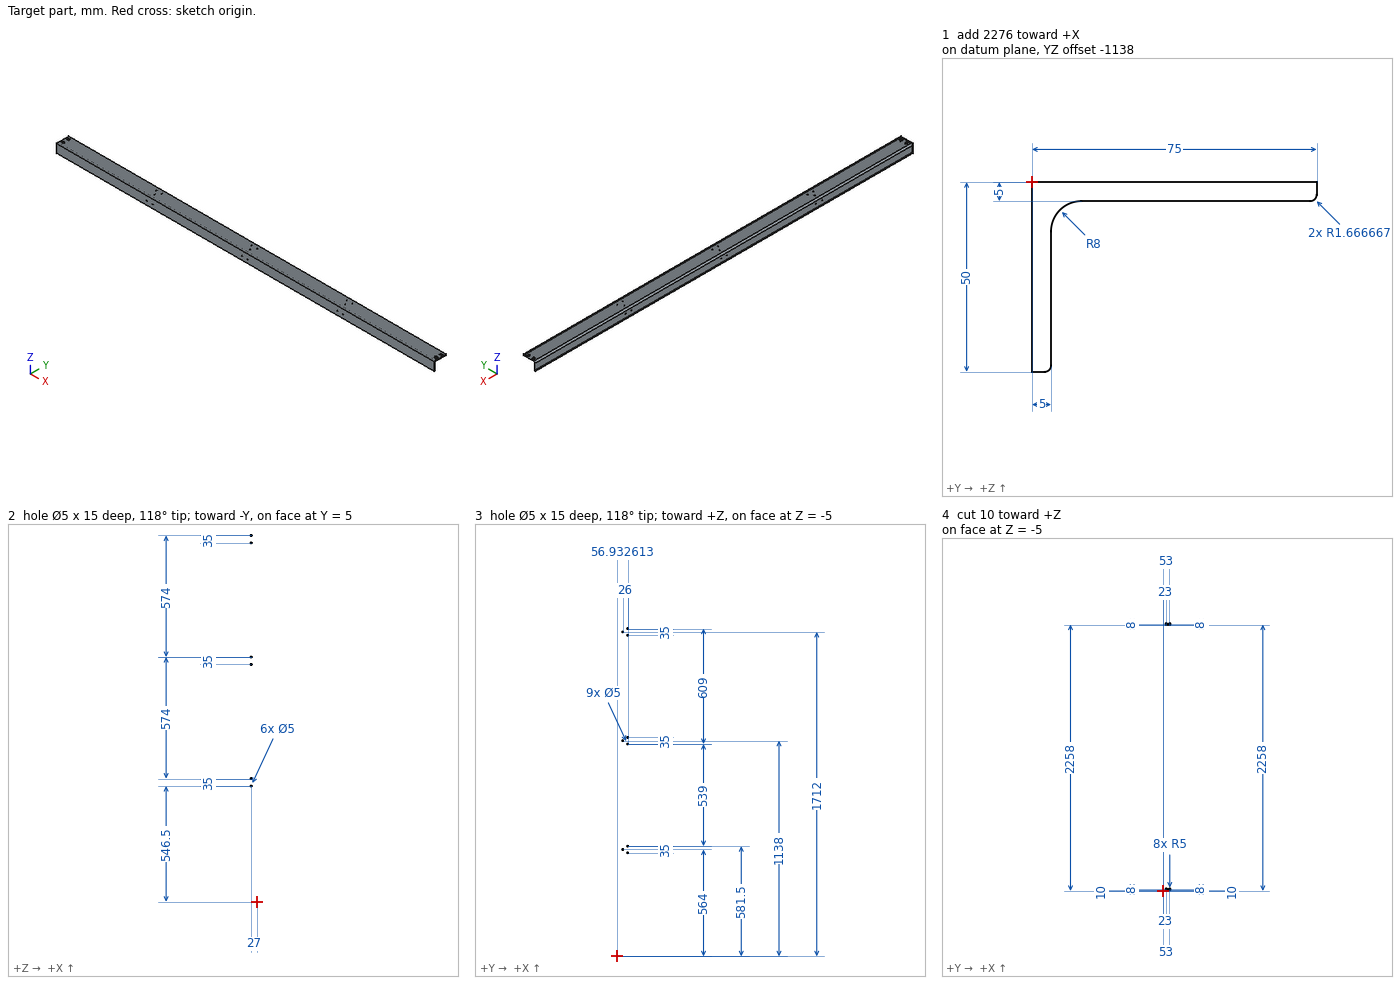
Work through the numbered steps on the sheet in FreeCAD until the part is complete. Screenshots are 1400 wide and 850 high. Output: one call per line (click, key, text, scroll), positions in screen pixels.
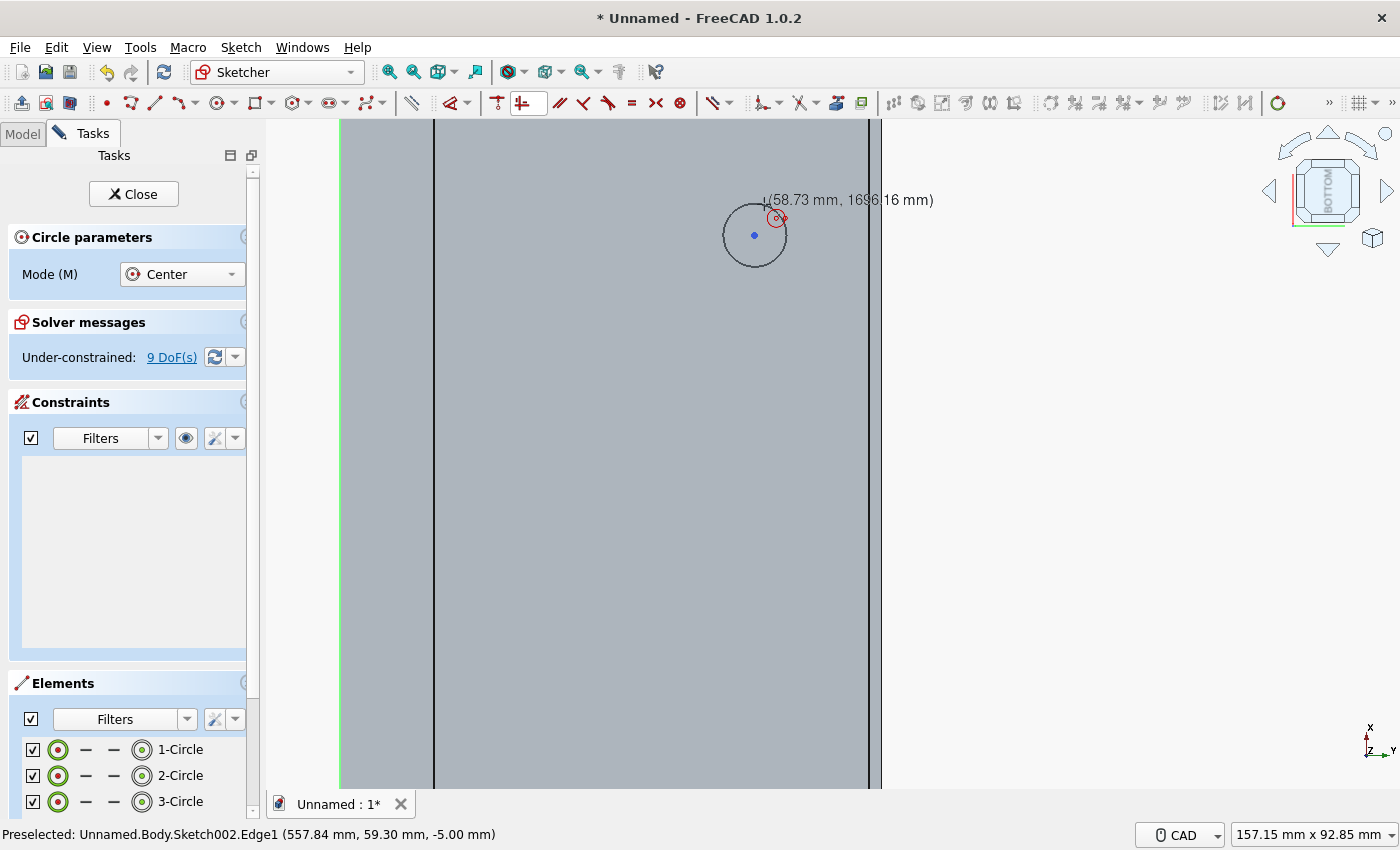
scroll(773, 210, down, 16)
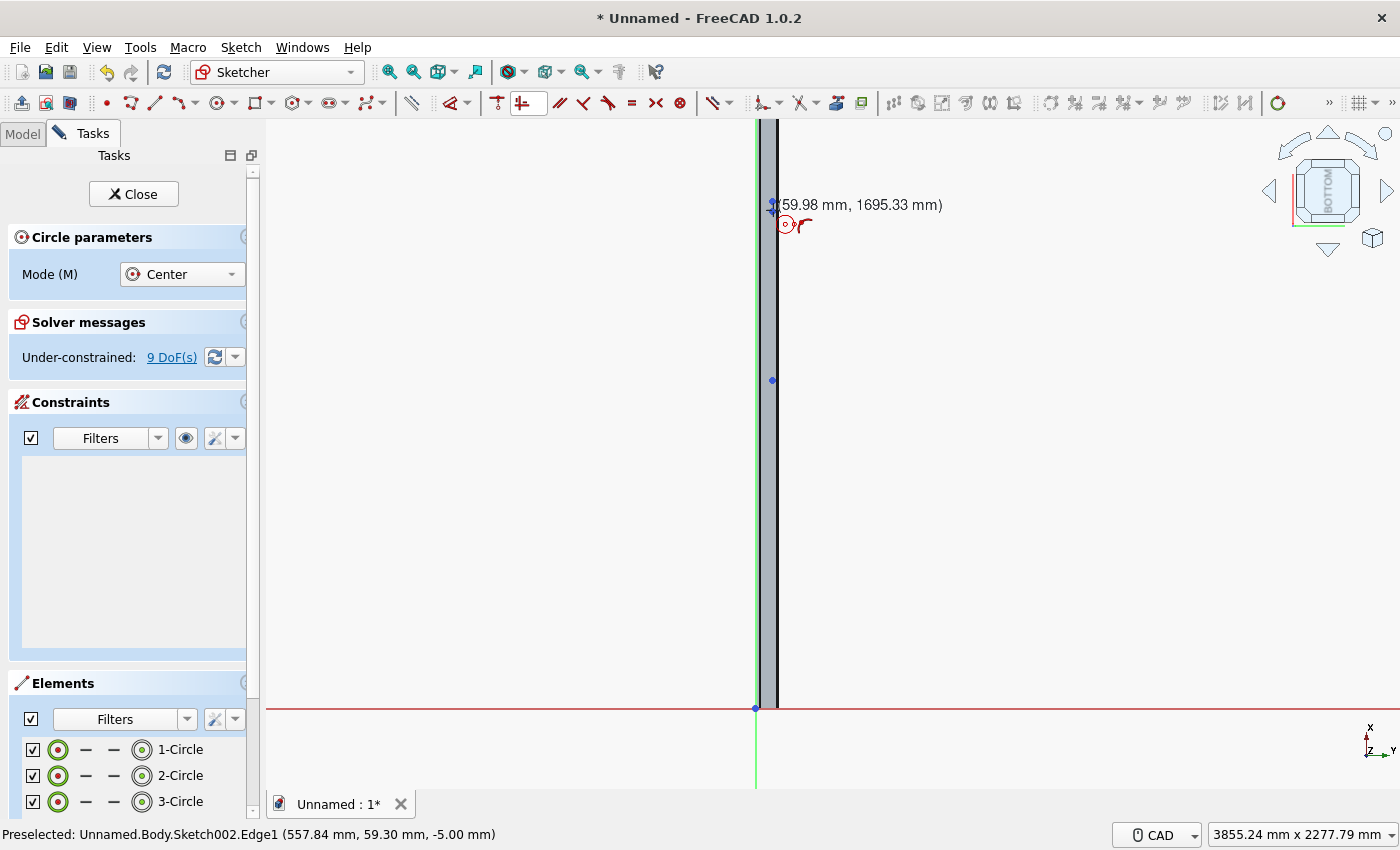
scroll(765, 205, up, 18)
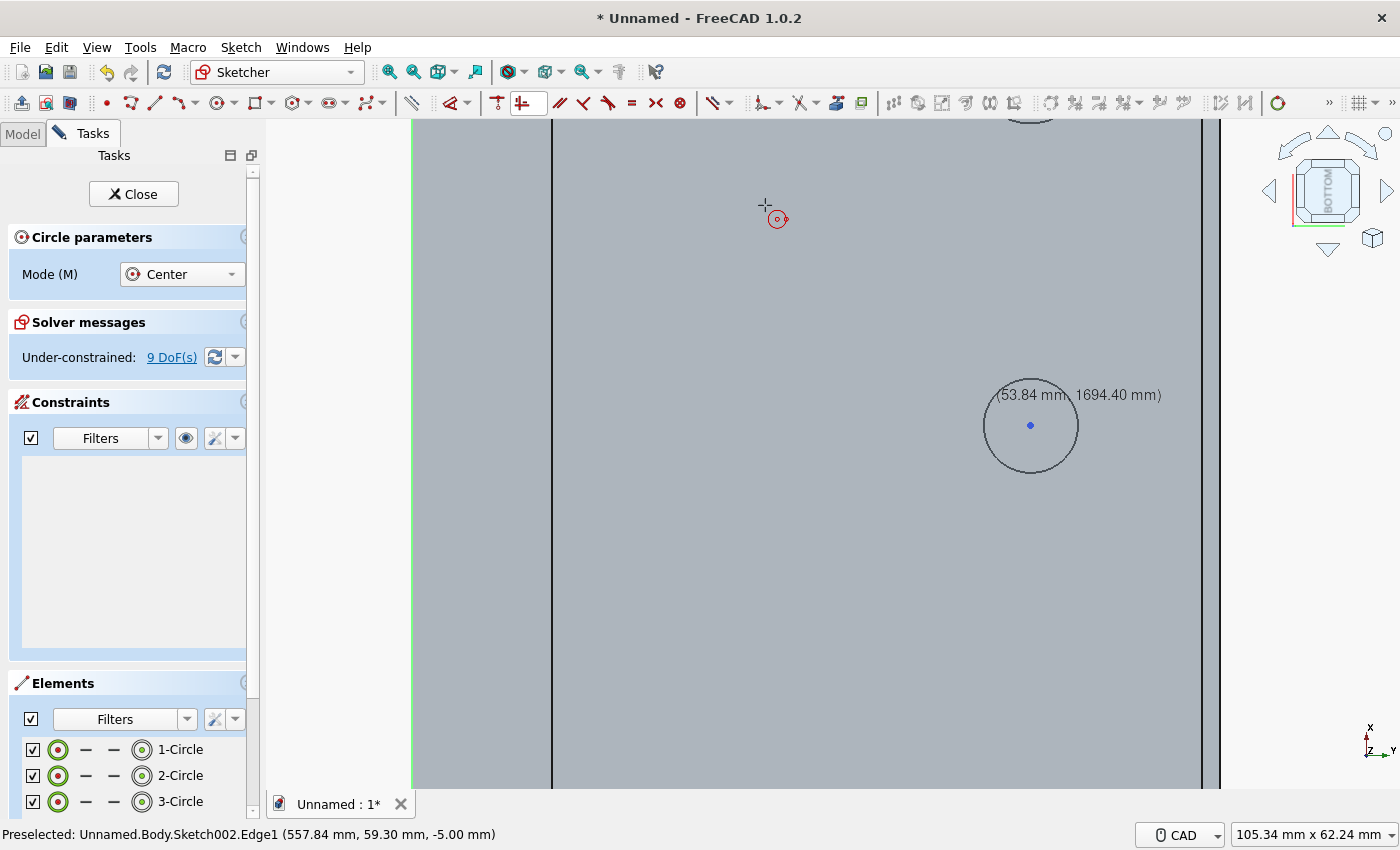
scroll(765, 205, down, 18)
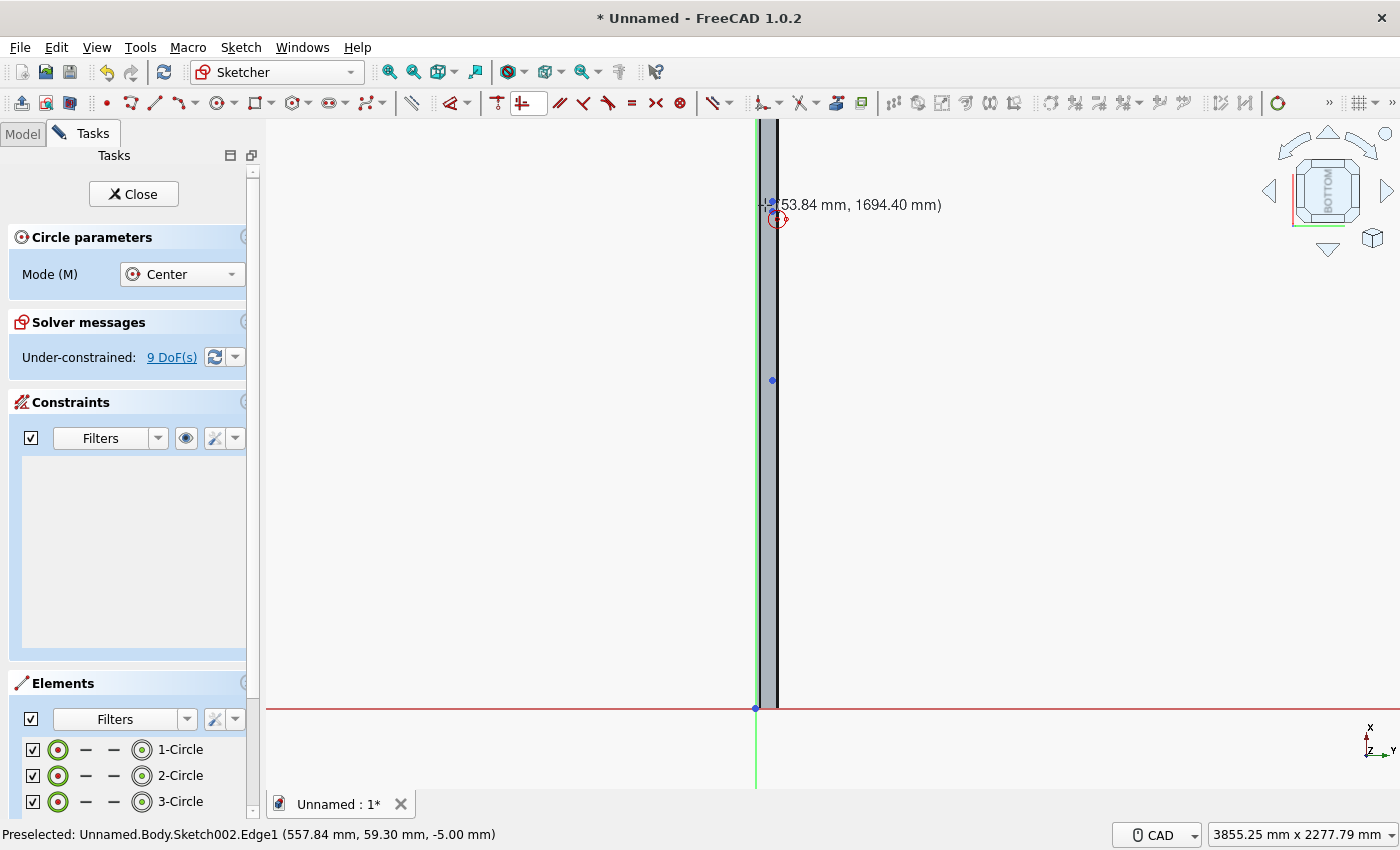
scroll(765, 205, up, 4)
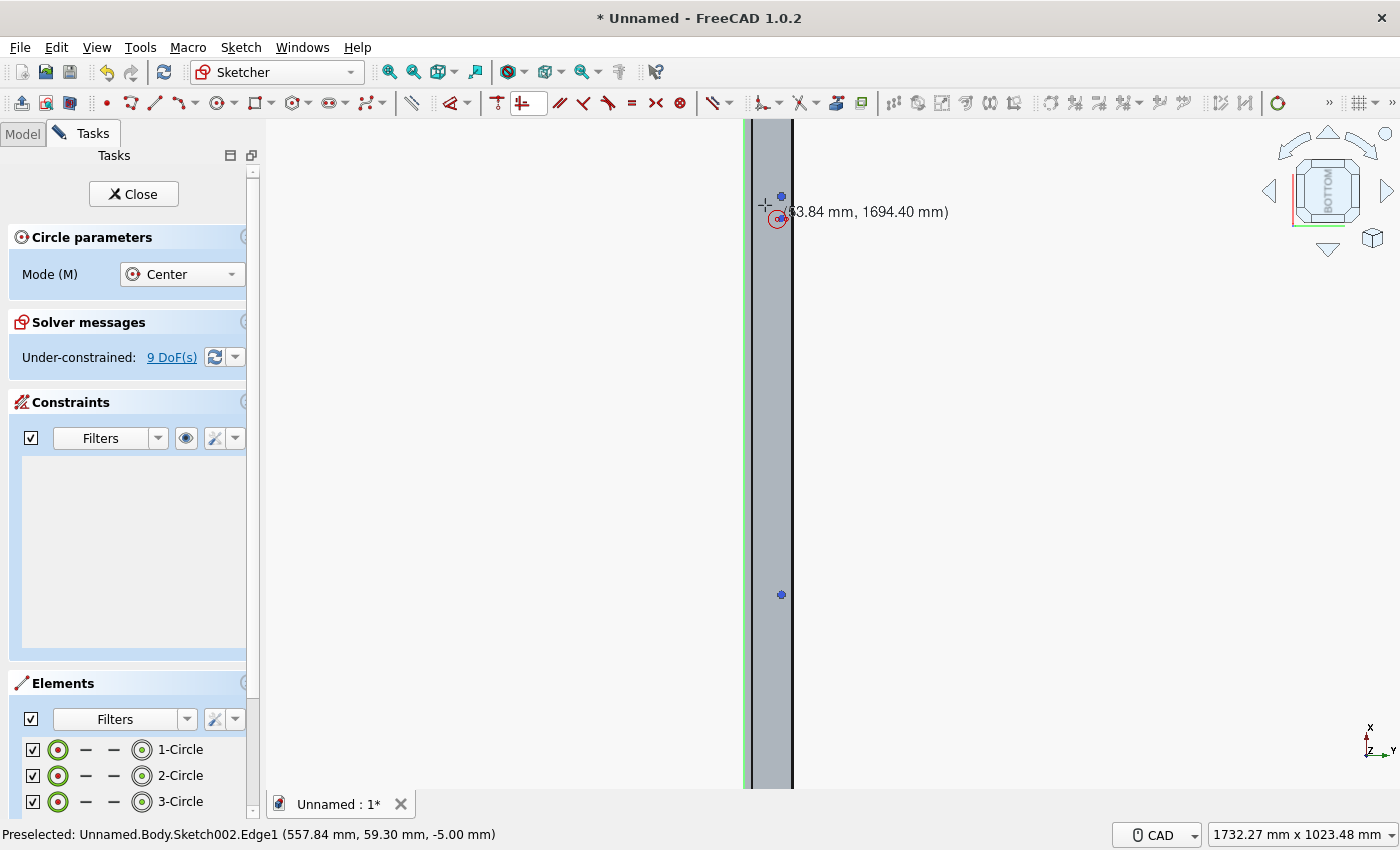
click(764, 205)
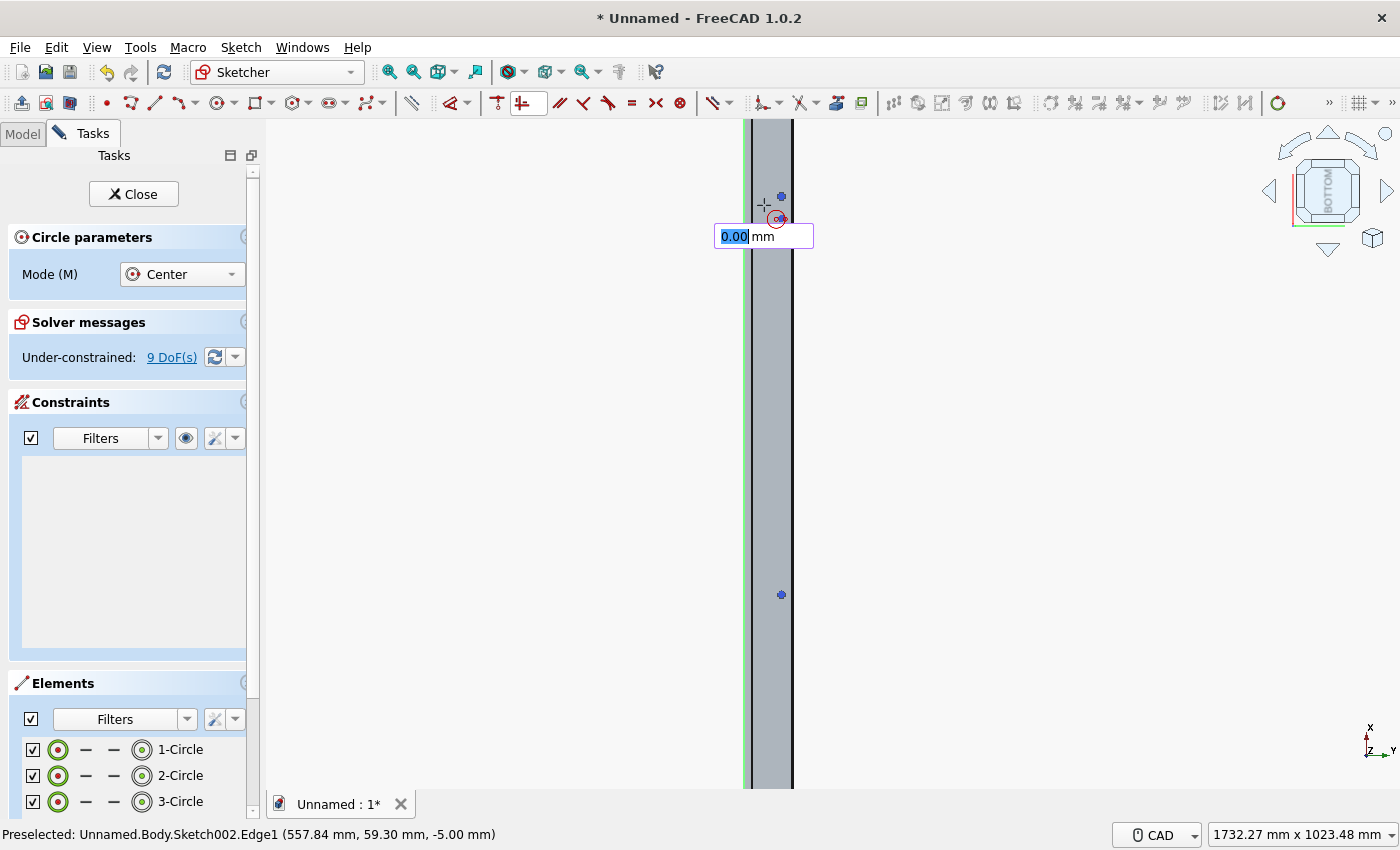
scroll(765, 204, up, 12)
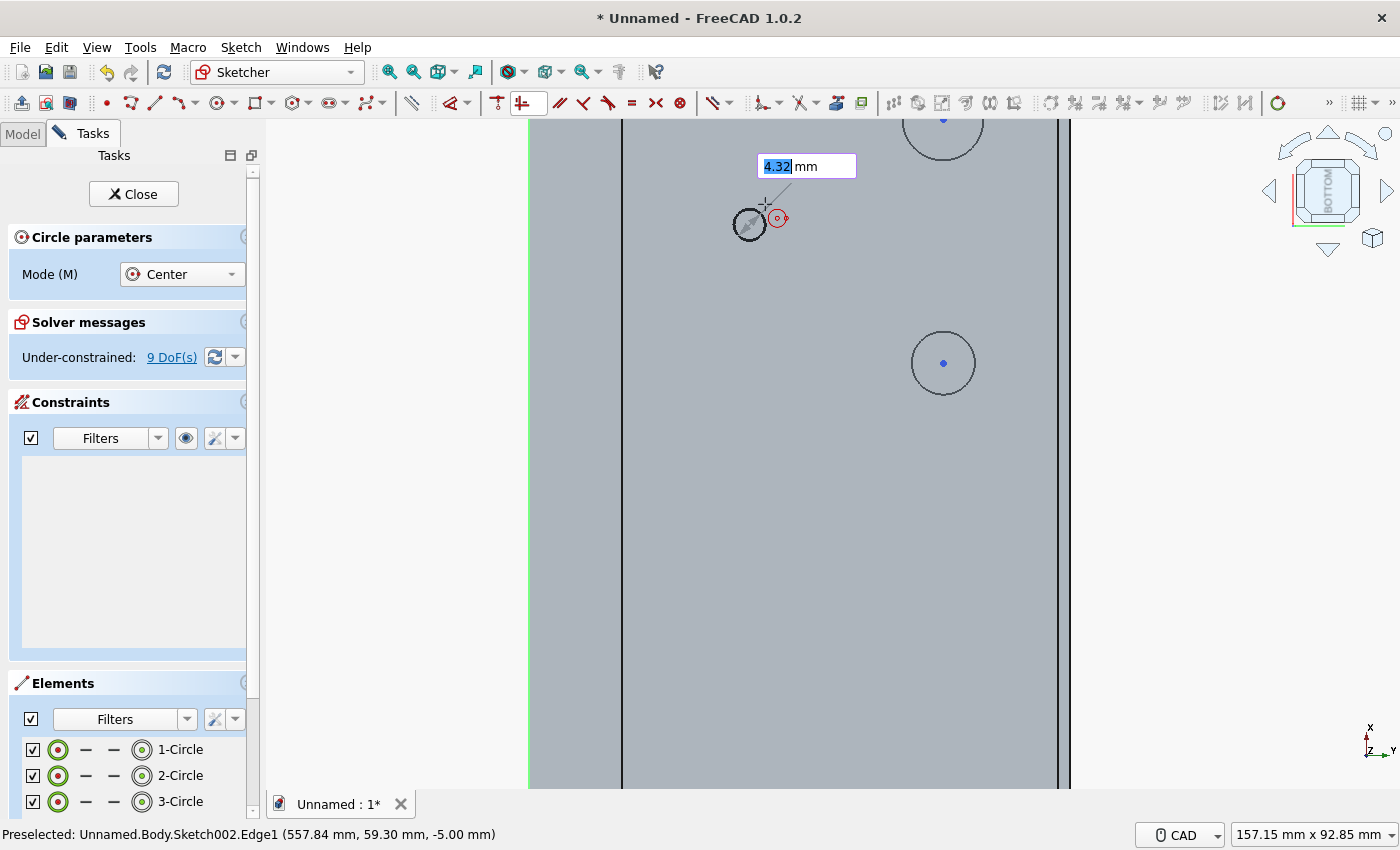
click(765, 206)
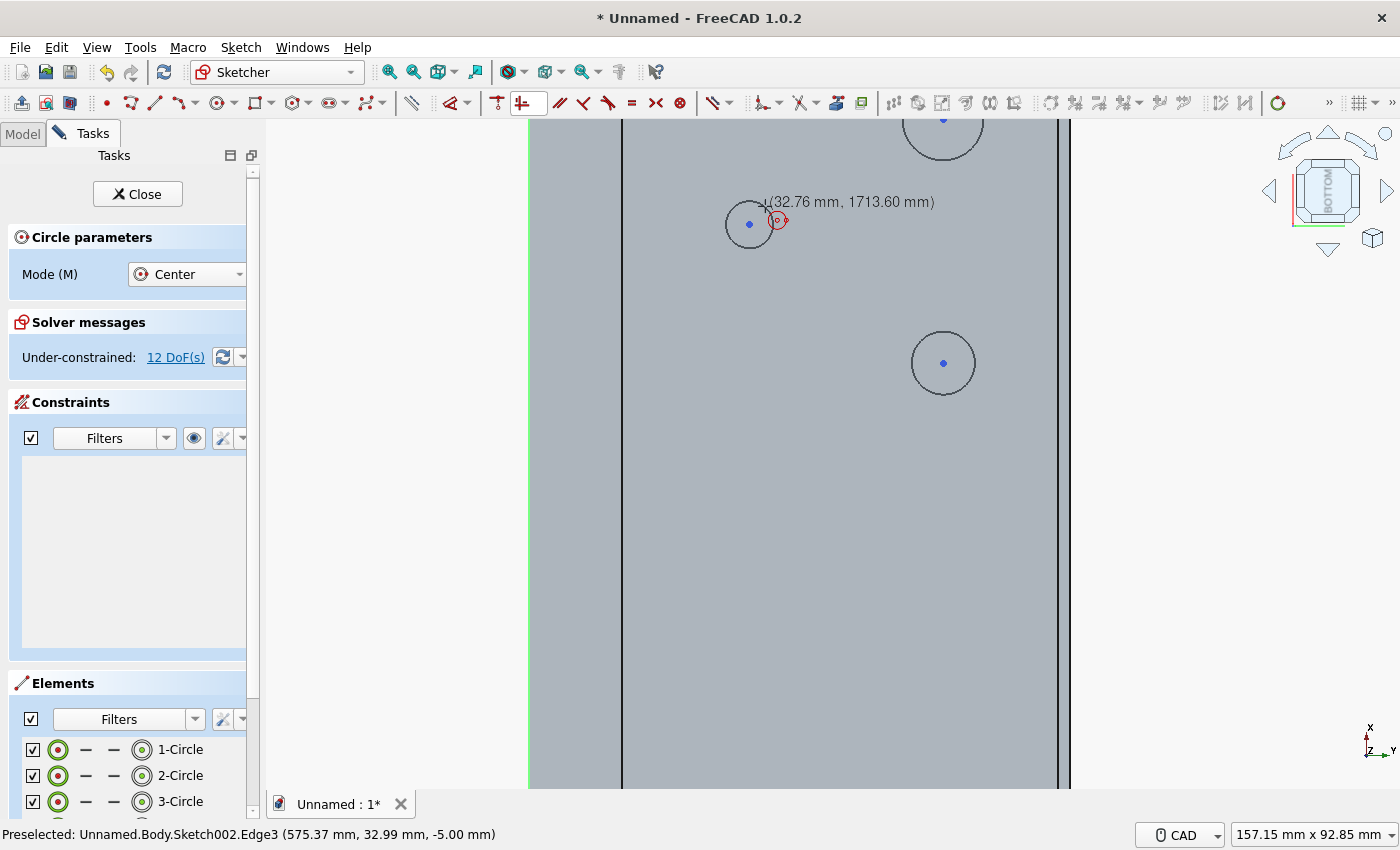
scroll(765, 205, down, 16)